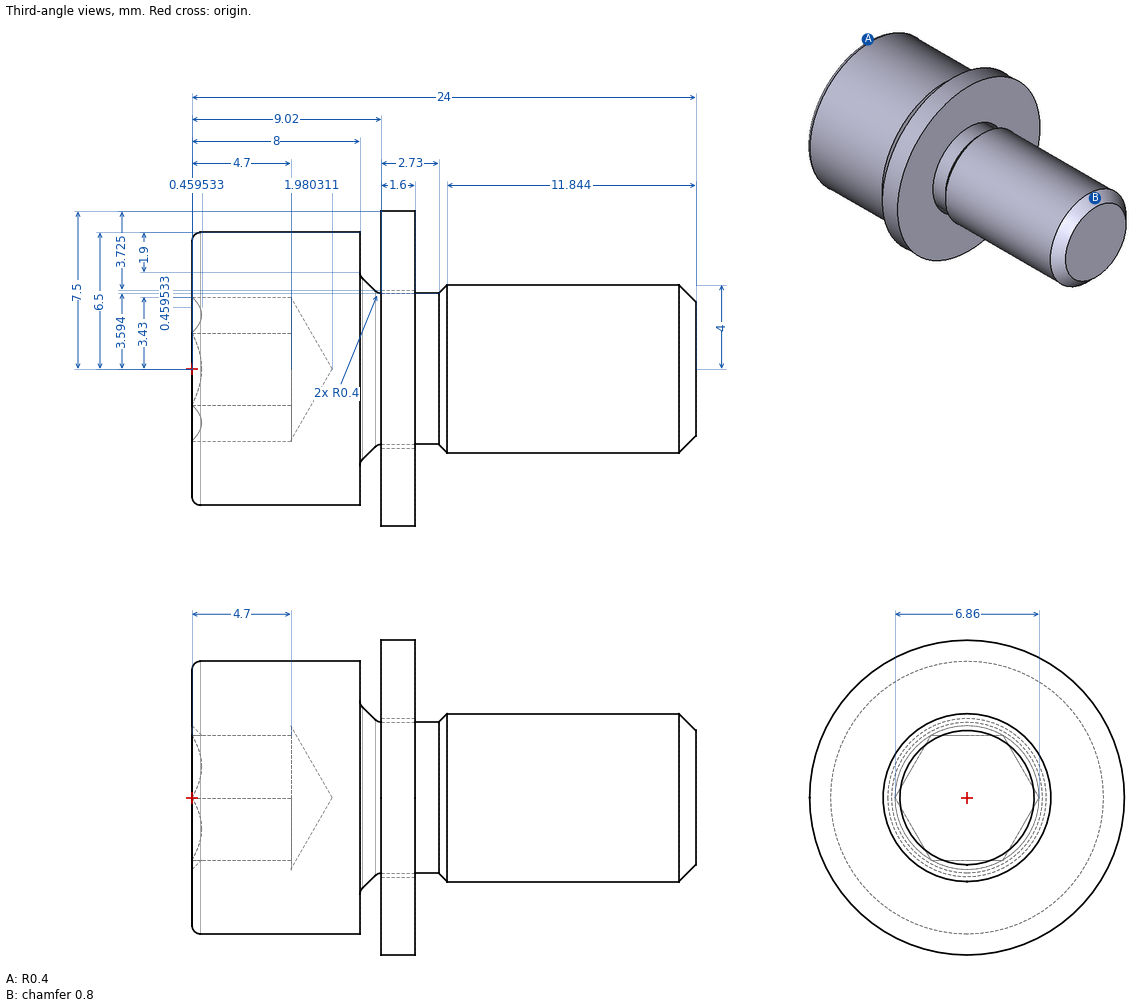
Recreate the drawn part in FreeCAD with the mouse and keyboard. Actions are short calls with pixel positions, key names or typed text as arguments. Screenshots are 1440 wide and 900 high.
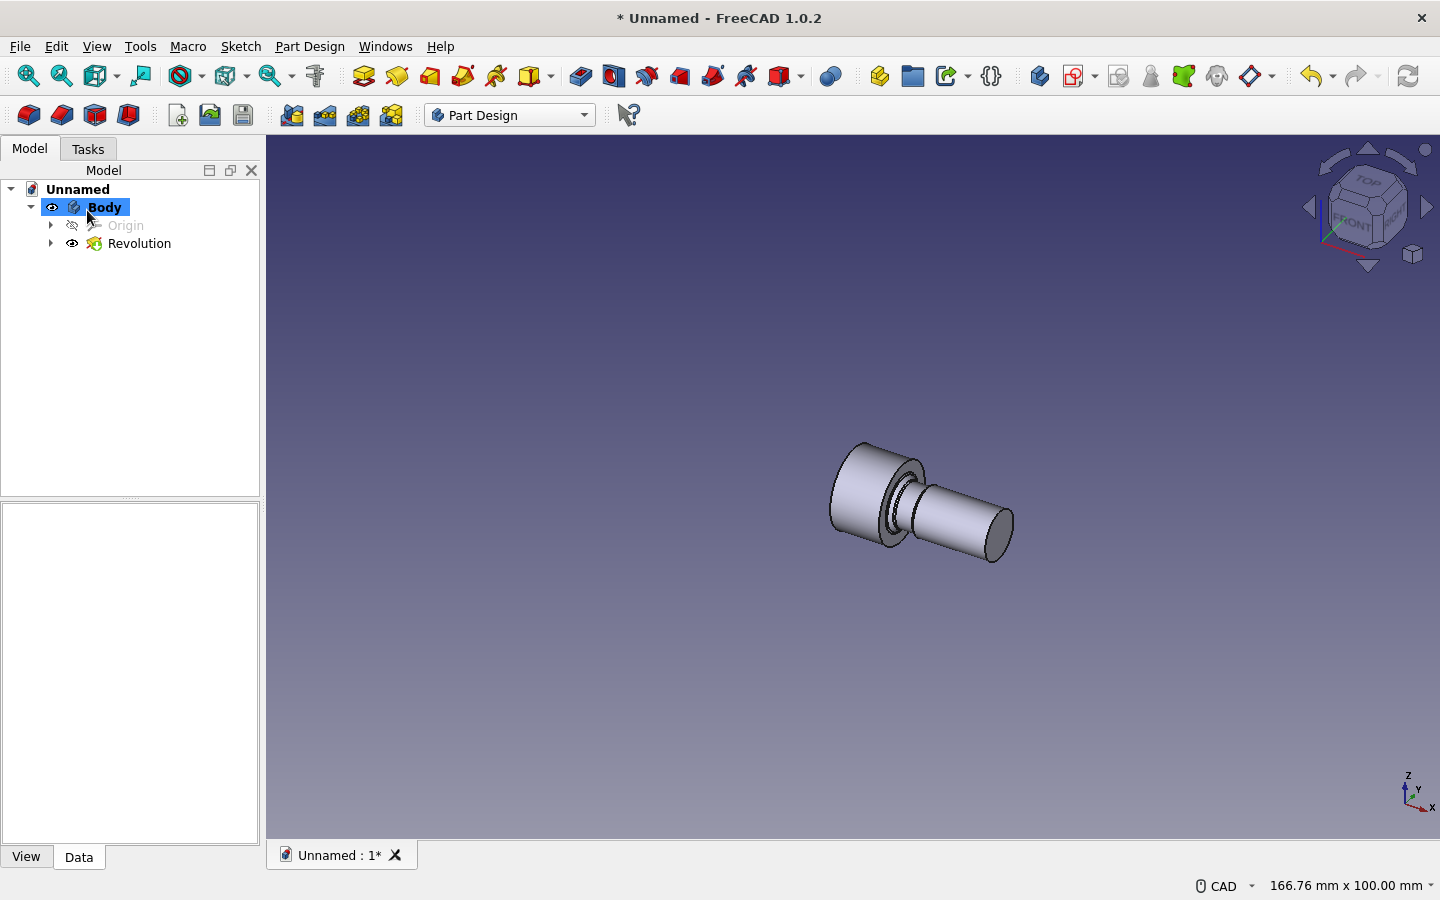
click(29, 76)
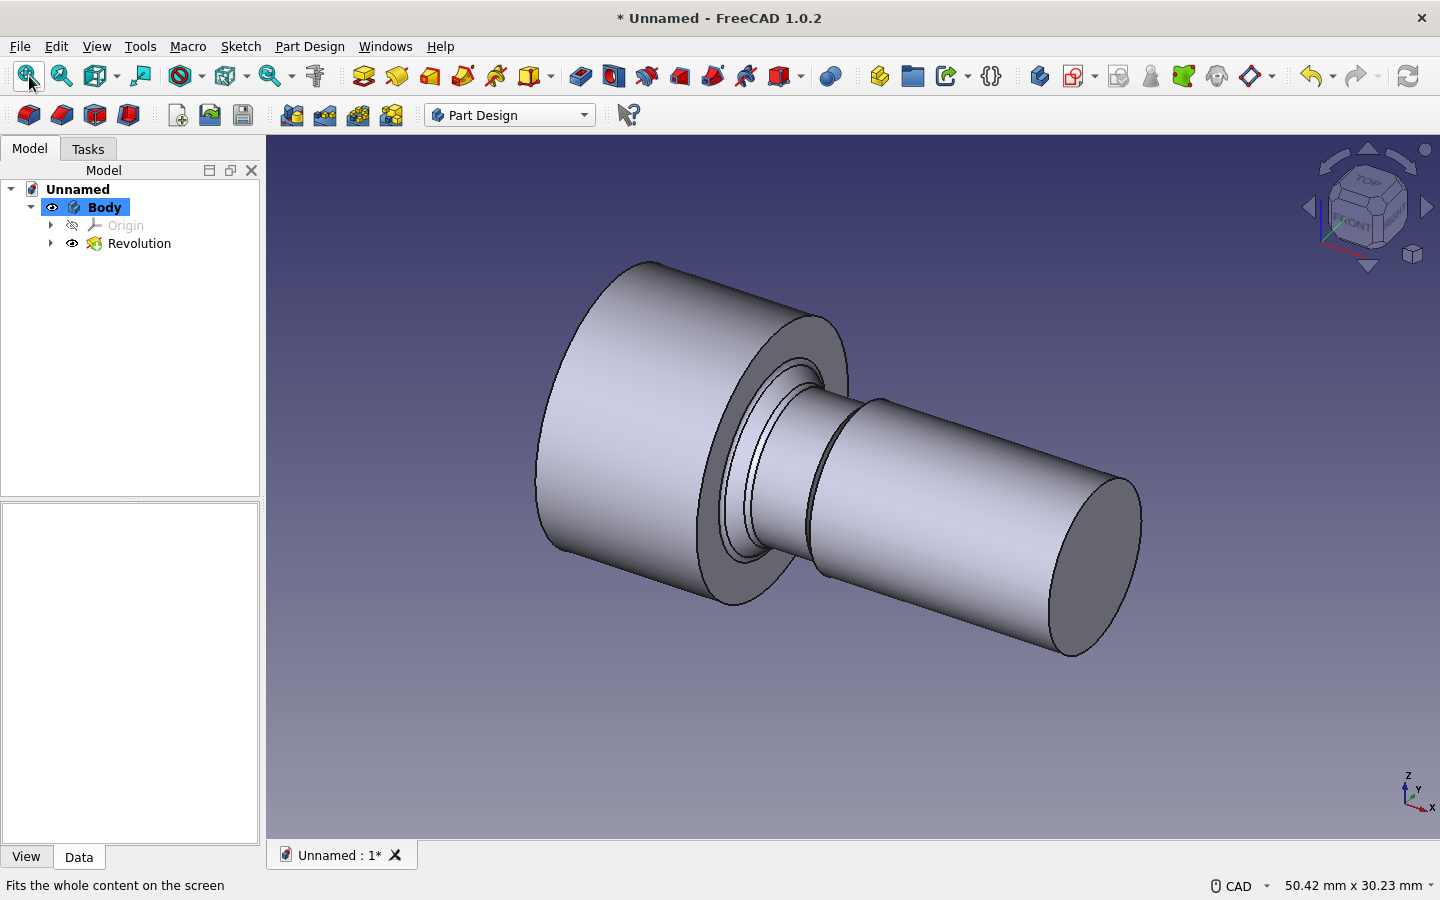
click(1072, 76)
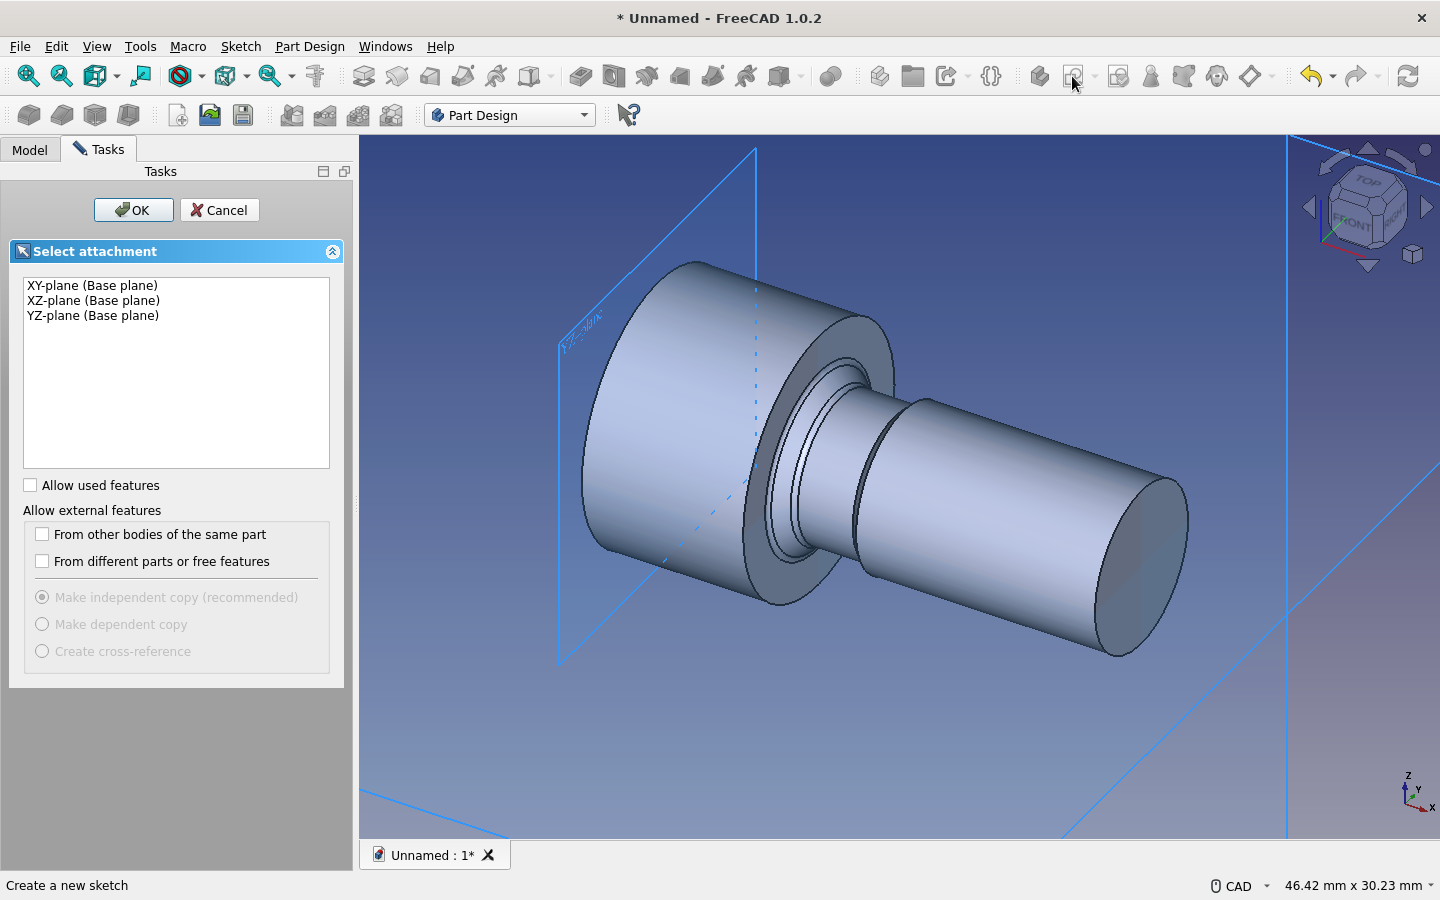
click(84, 316)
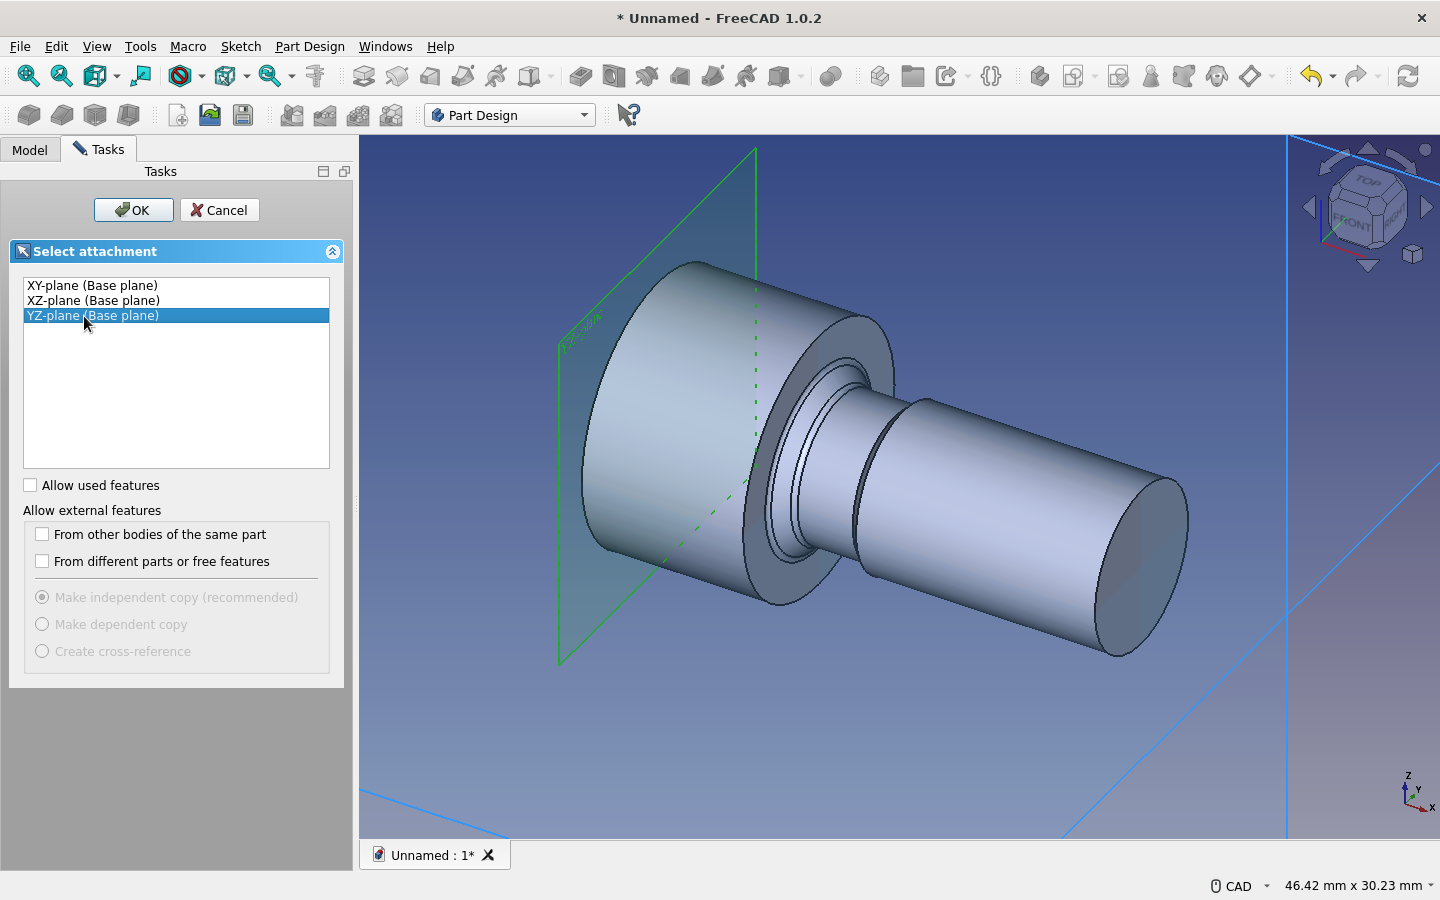
click(134, 210)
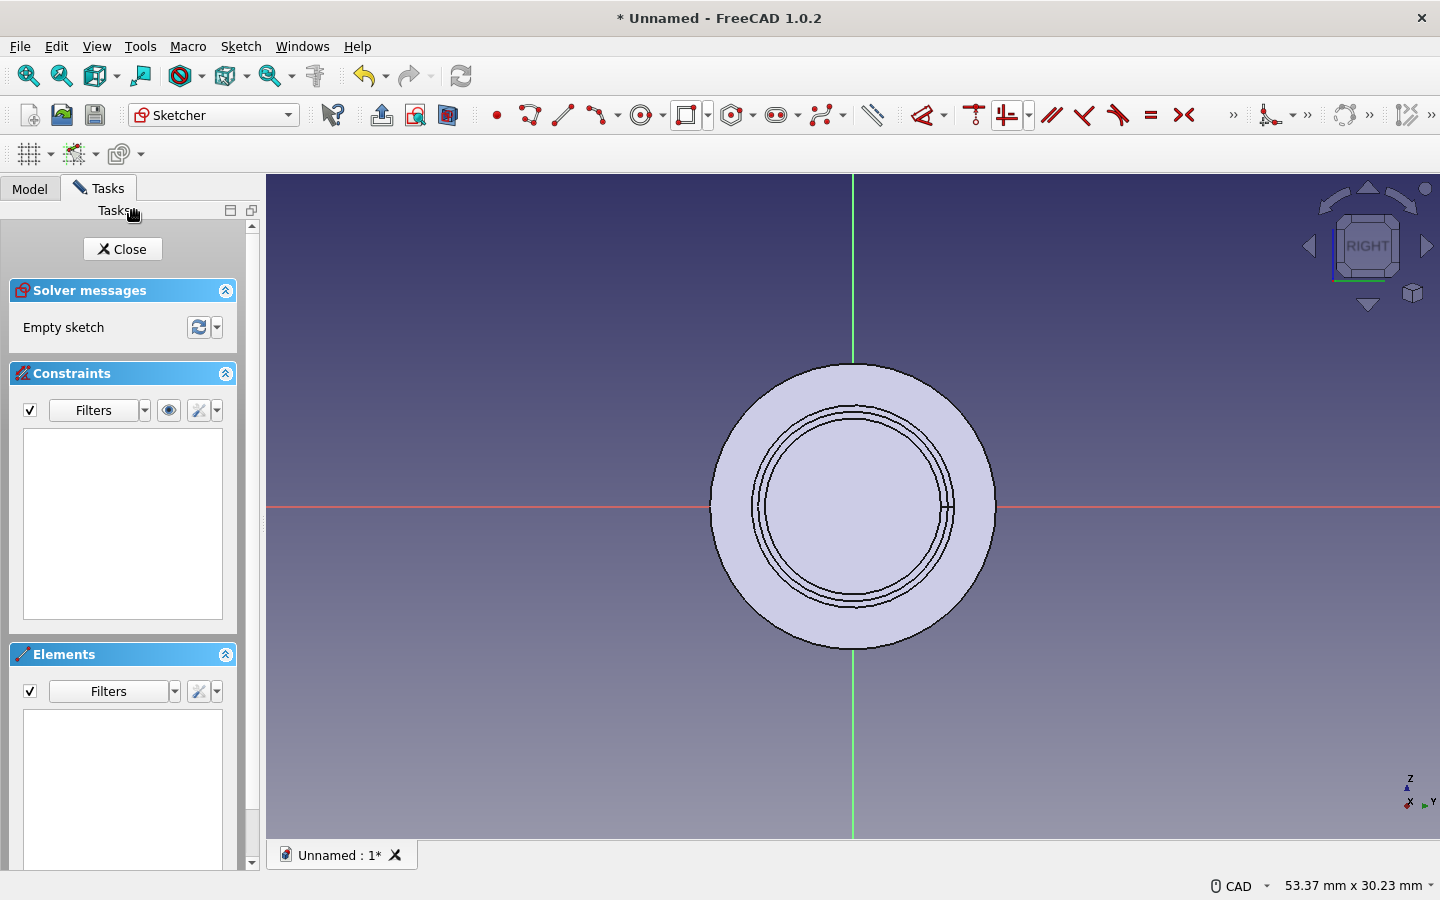
click(448, 116)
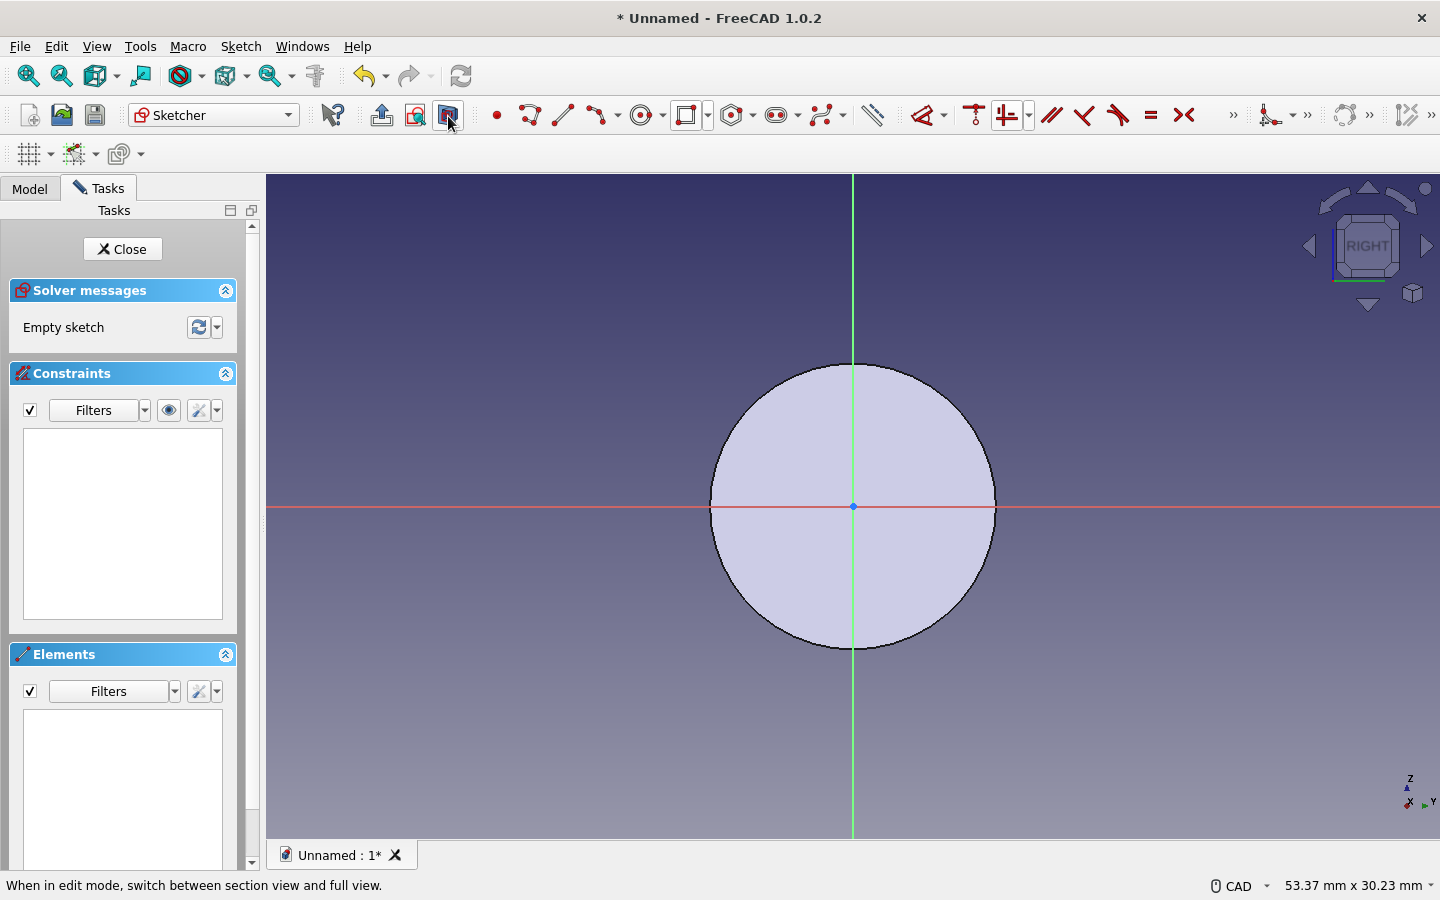
scroll(883, 506, up, 6)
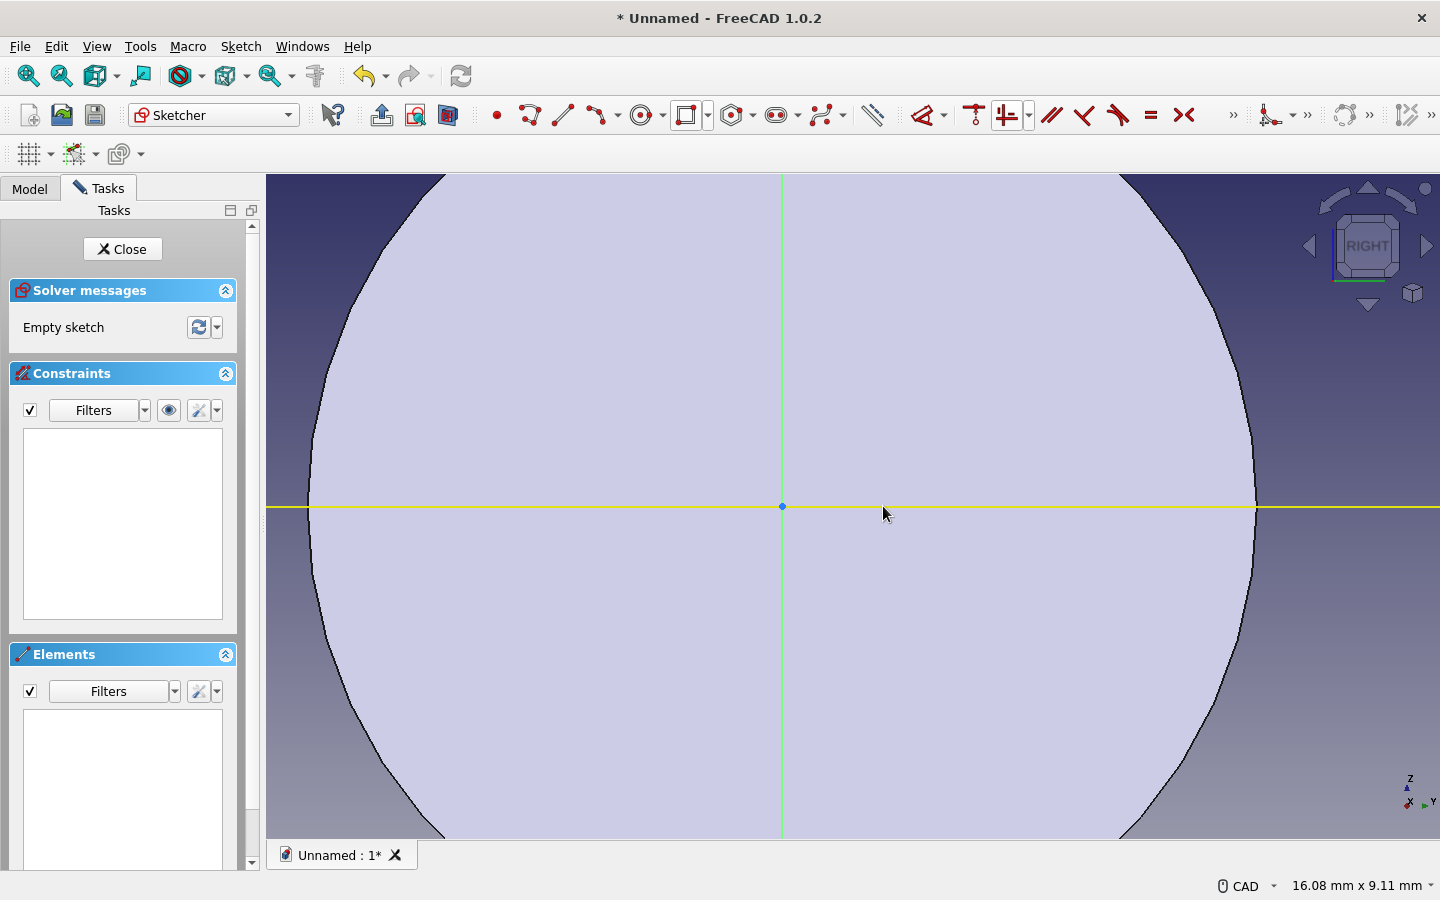
click(730, 116)